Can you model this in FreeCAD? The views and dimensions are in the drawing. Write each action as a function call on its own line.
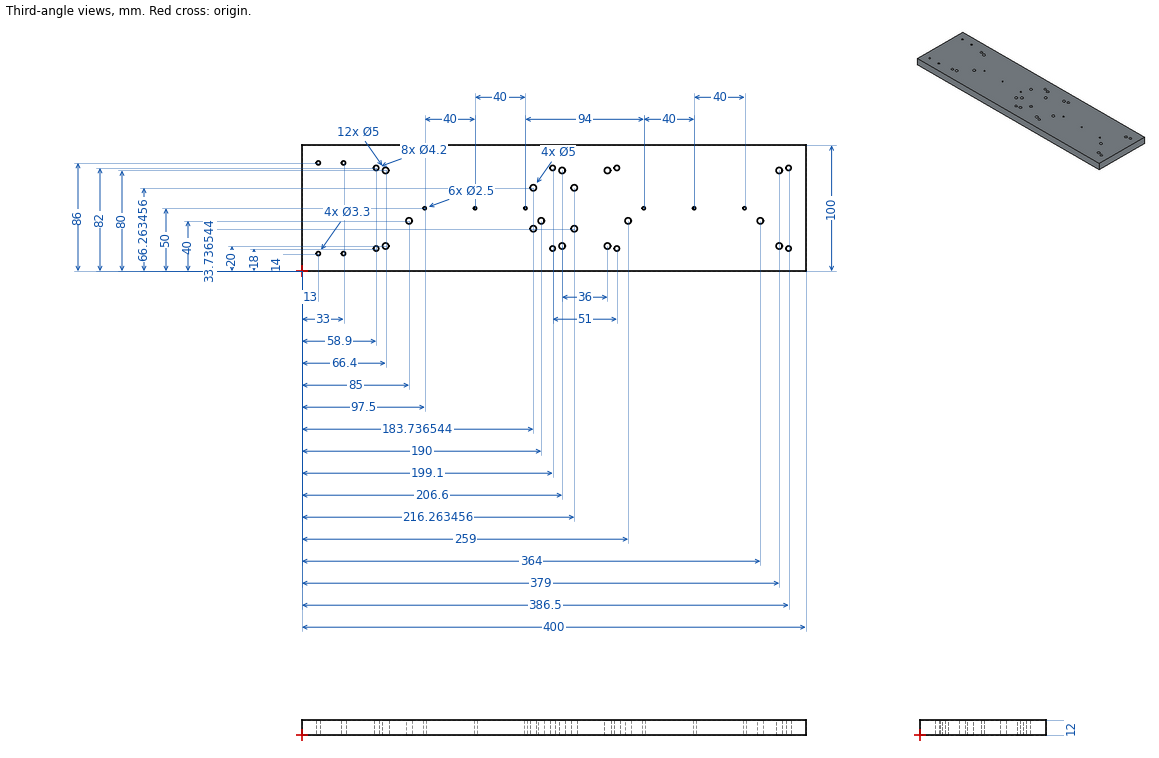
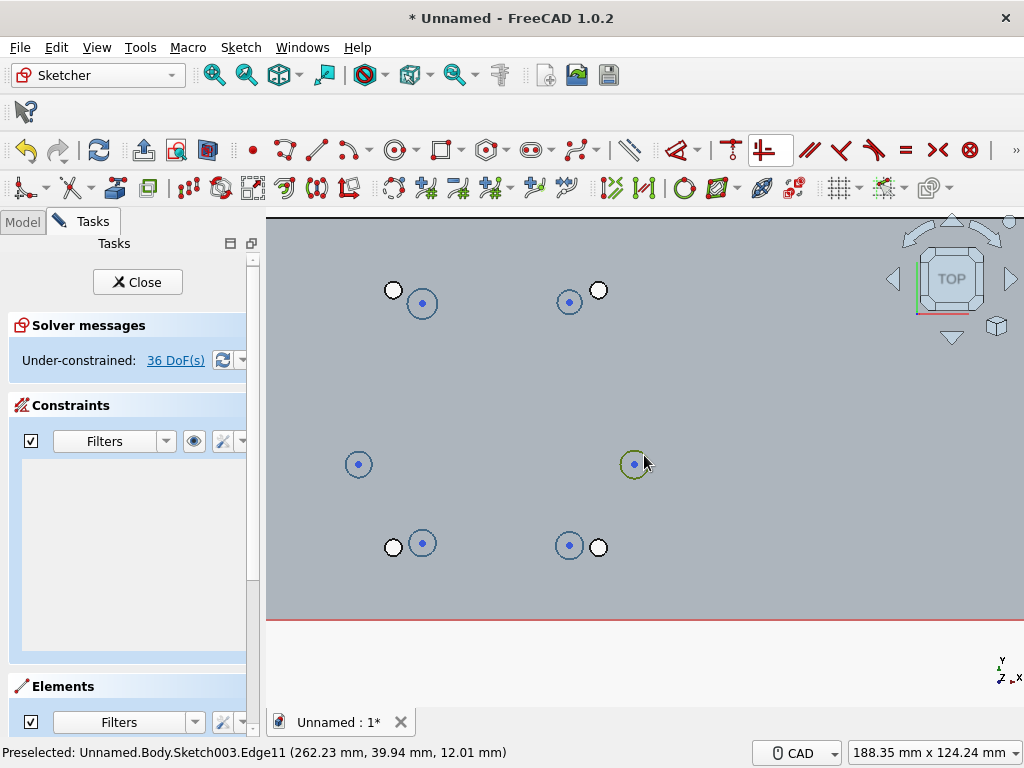
scroll(647, 458, down, 7)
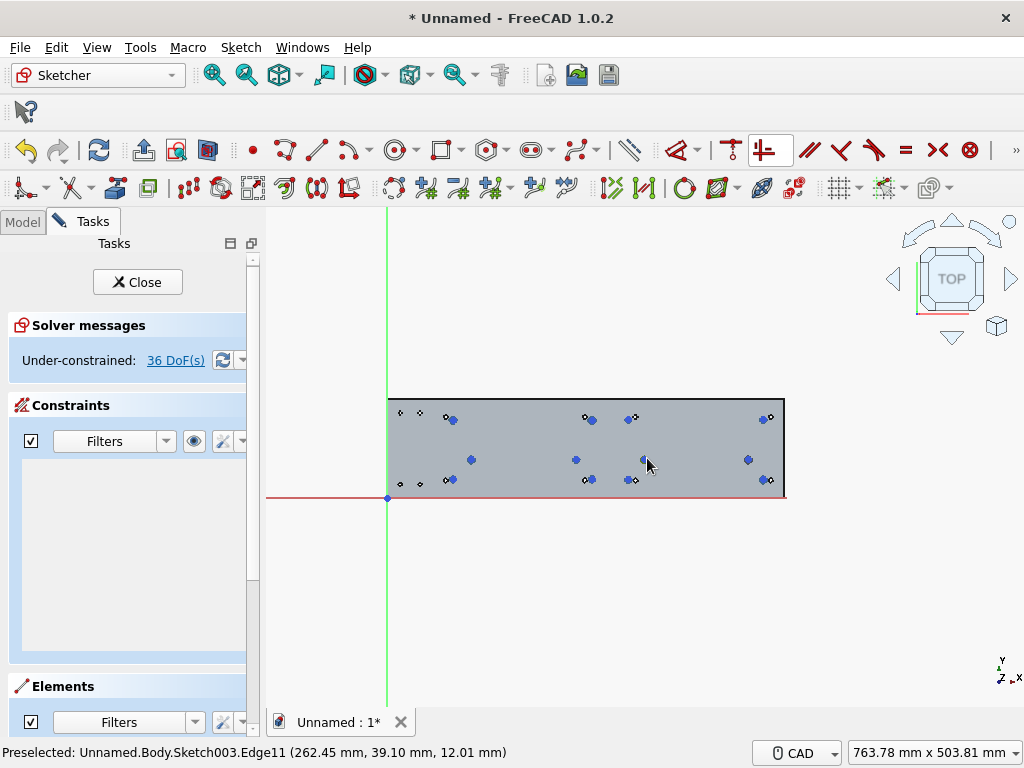
scroll(751, 457, up, 7)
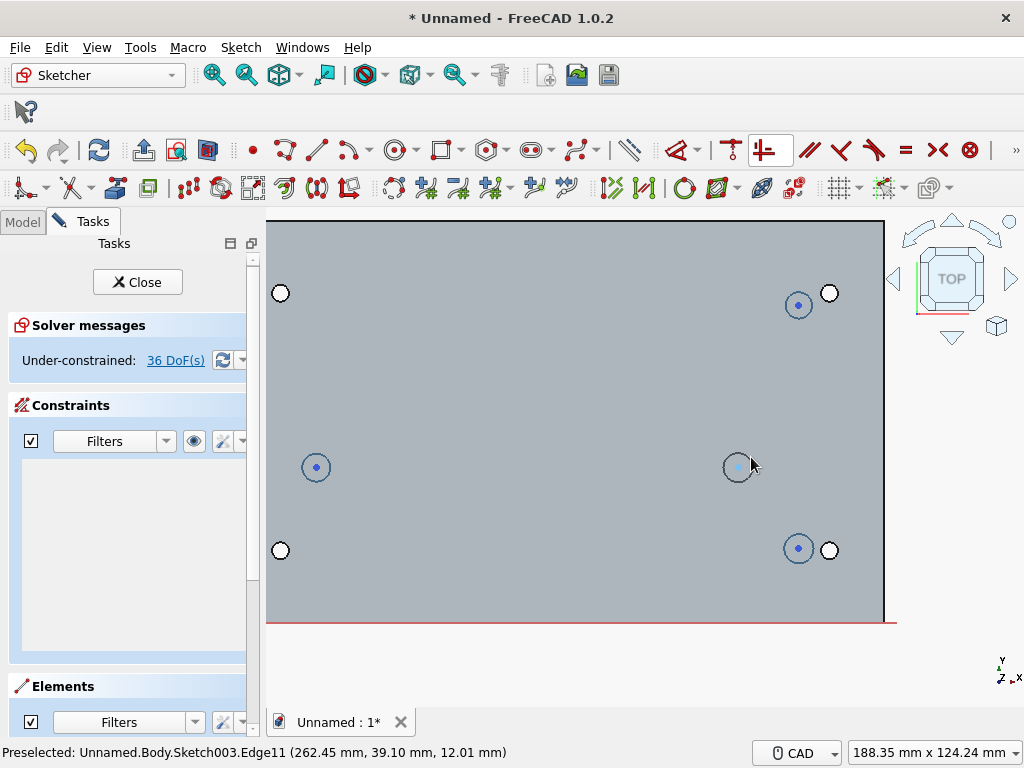
click(748, 457)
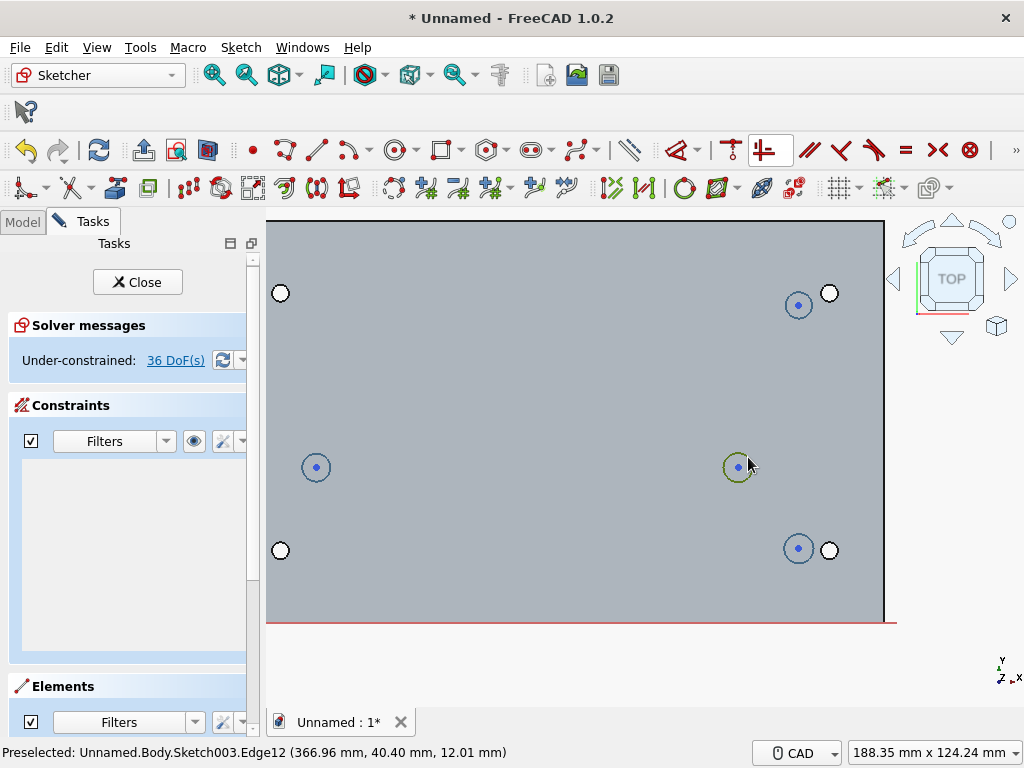
click(906, 150)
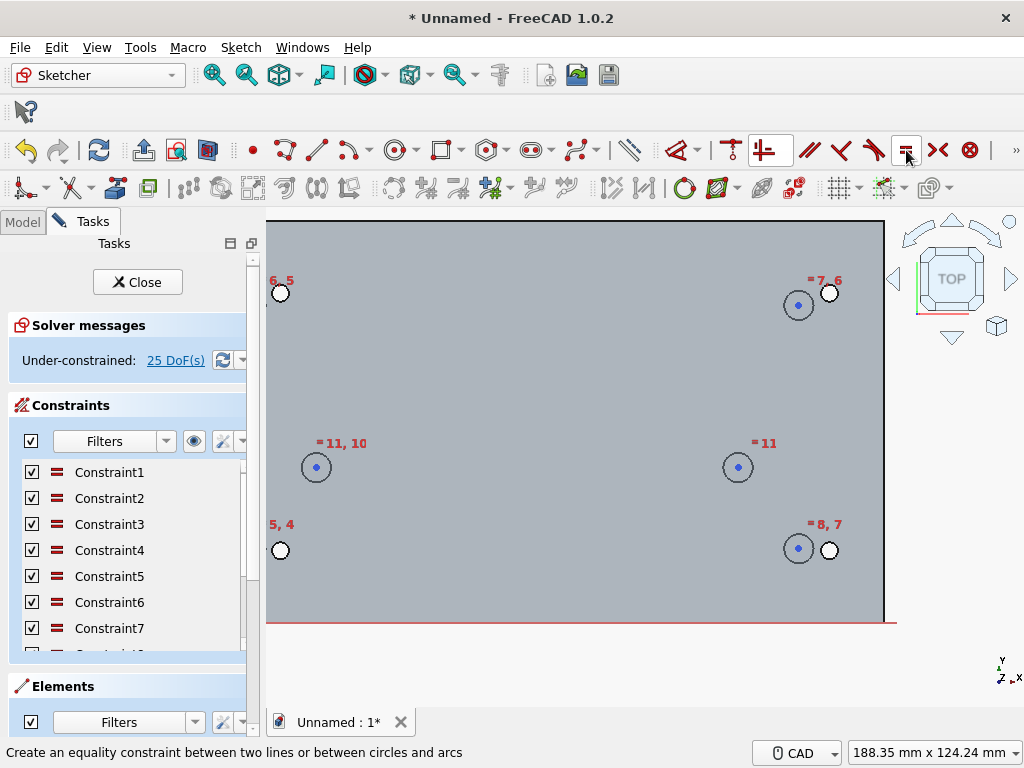
scroll(752, 457, down, 7)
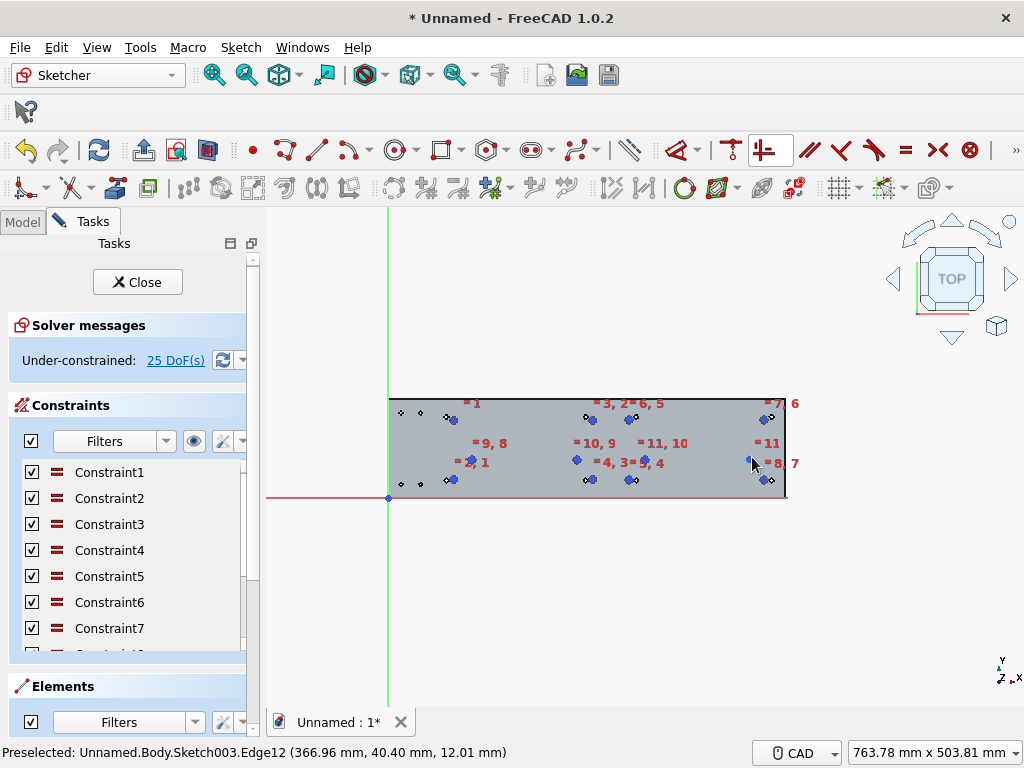
click(454, 420)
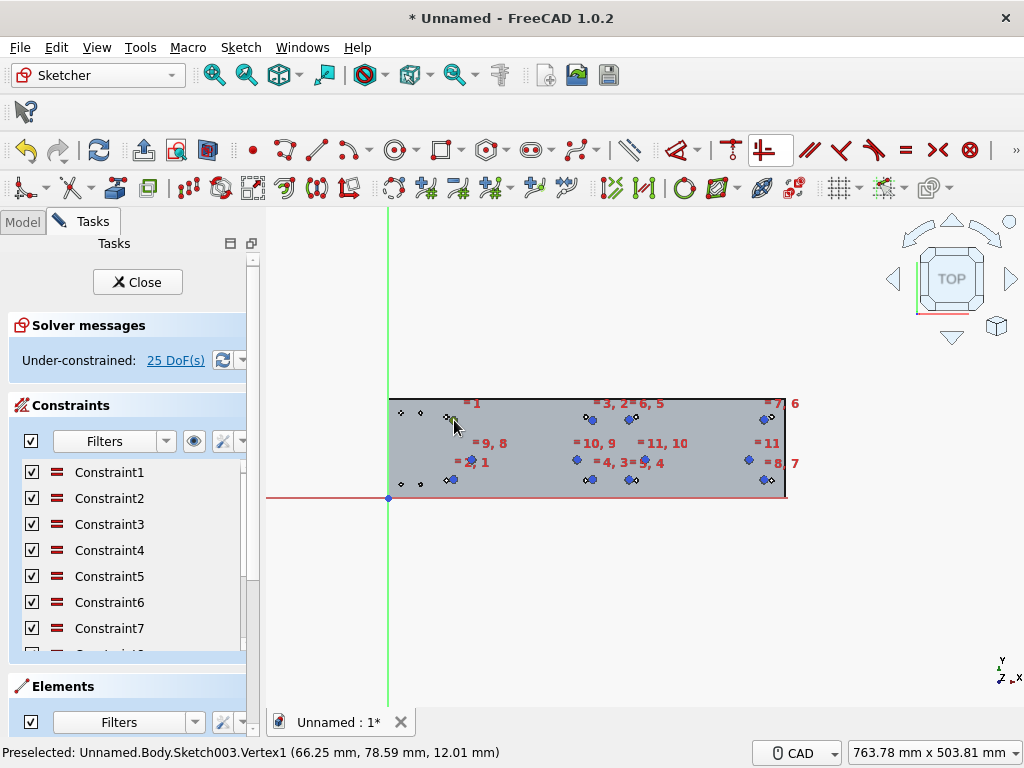
click(454, 479)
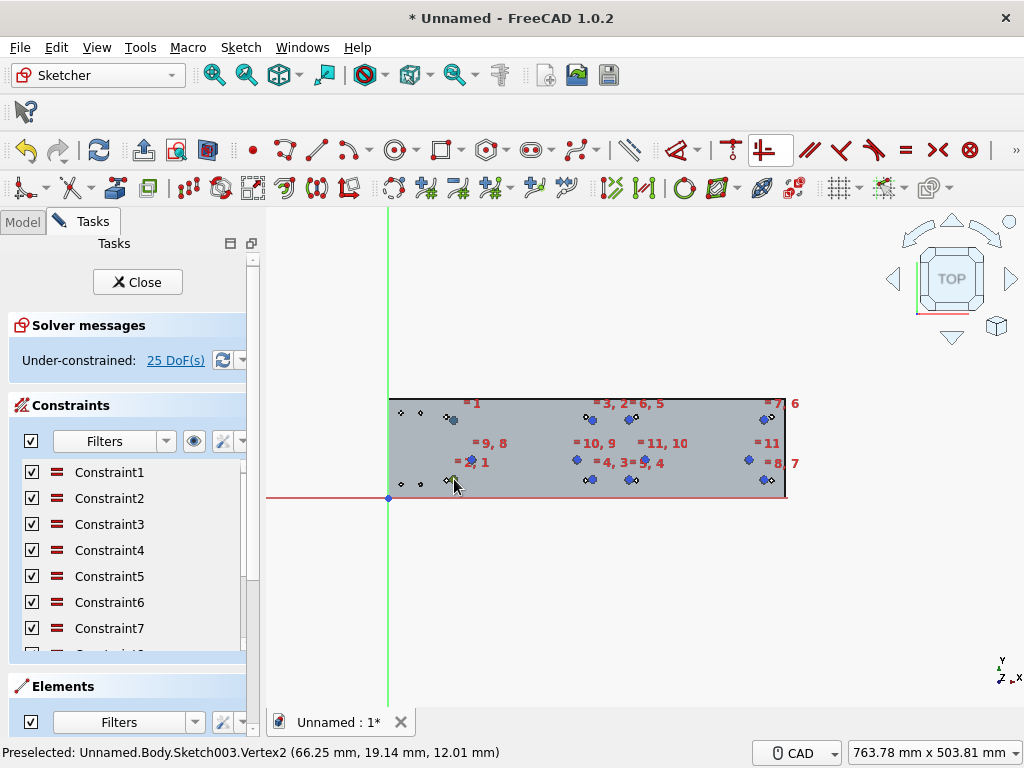
key(v)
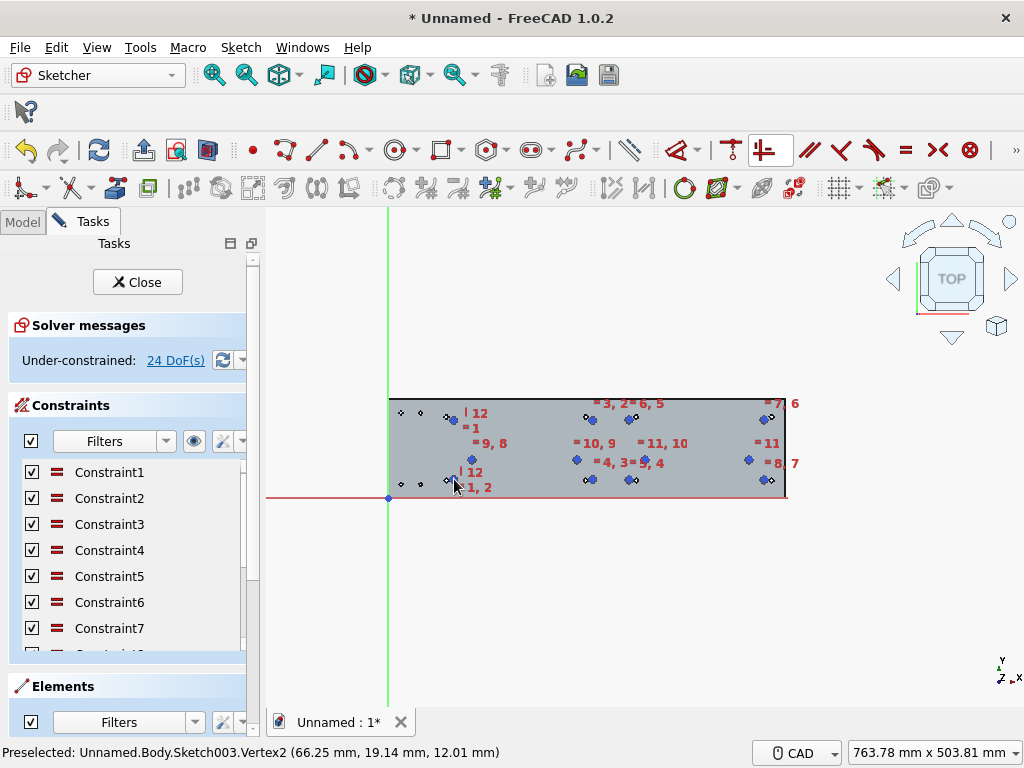
click(454, 420)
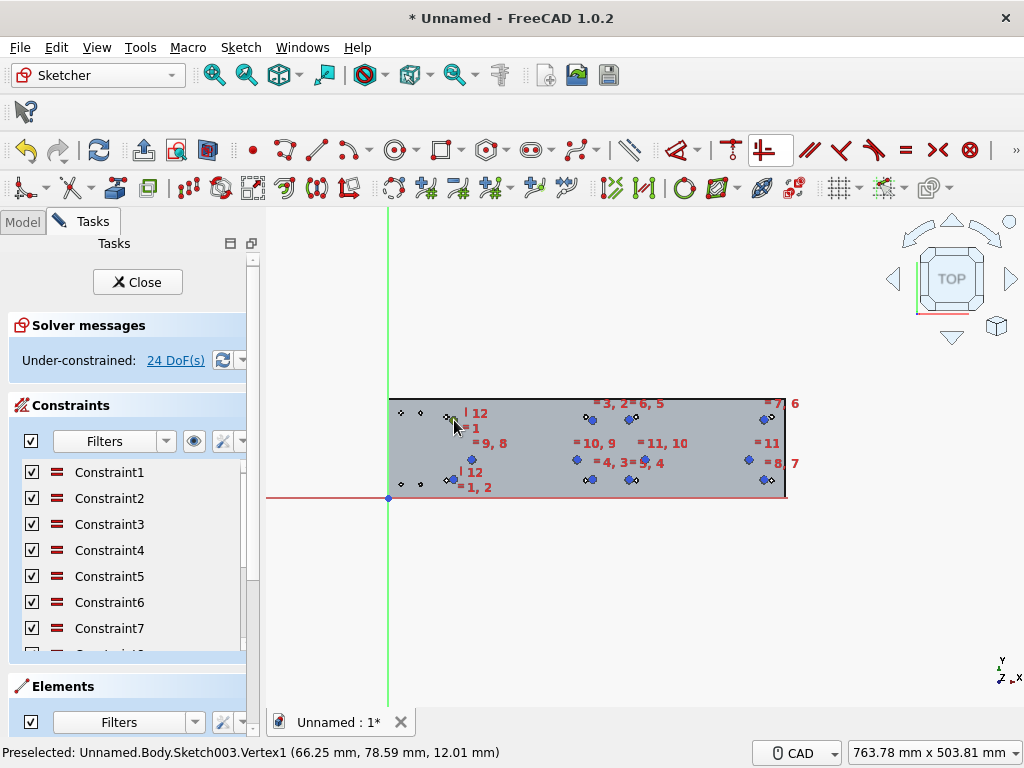
click(593, 420)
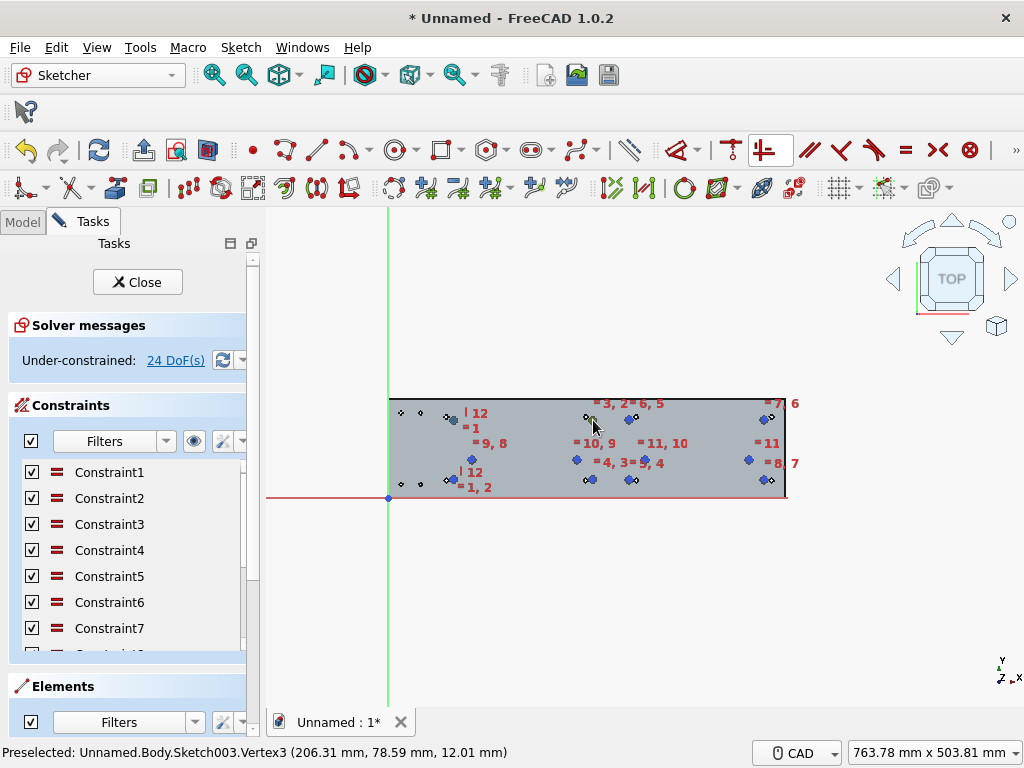
key(h)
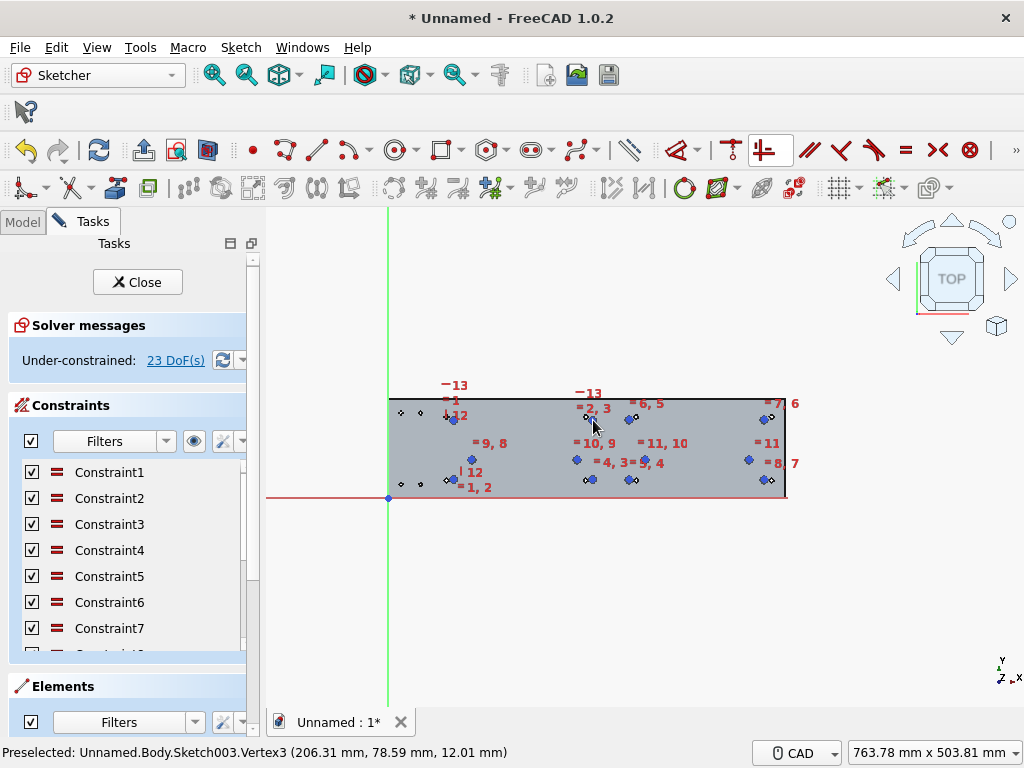
click(593, 420)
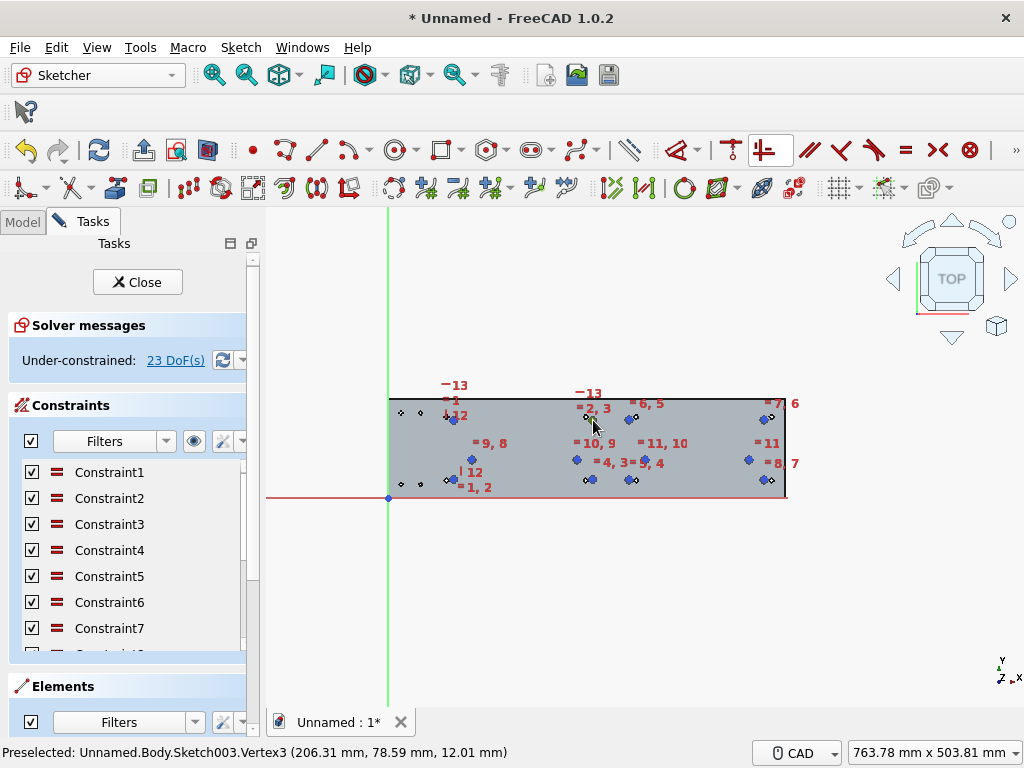
click(593, 479)